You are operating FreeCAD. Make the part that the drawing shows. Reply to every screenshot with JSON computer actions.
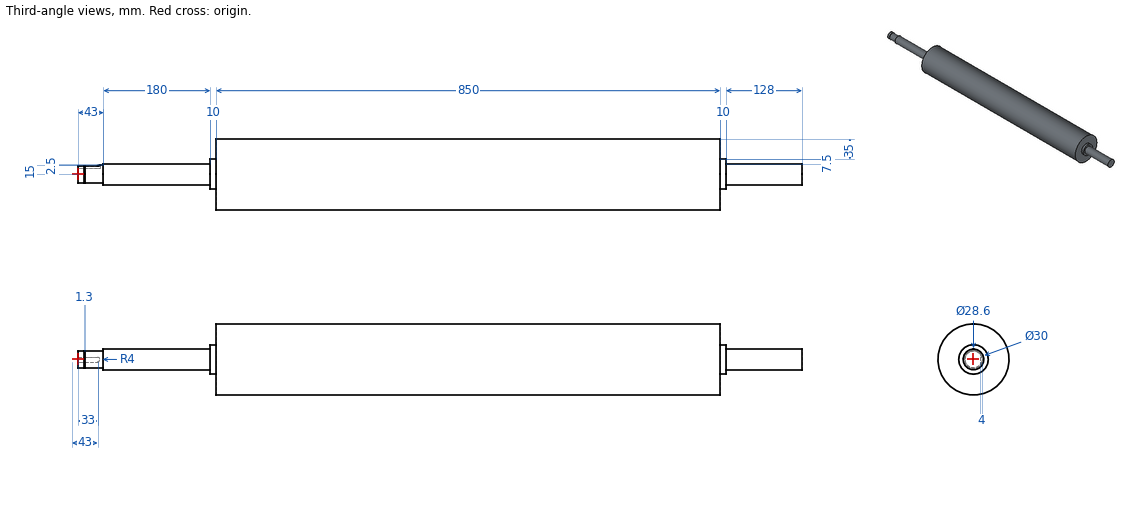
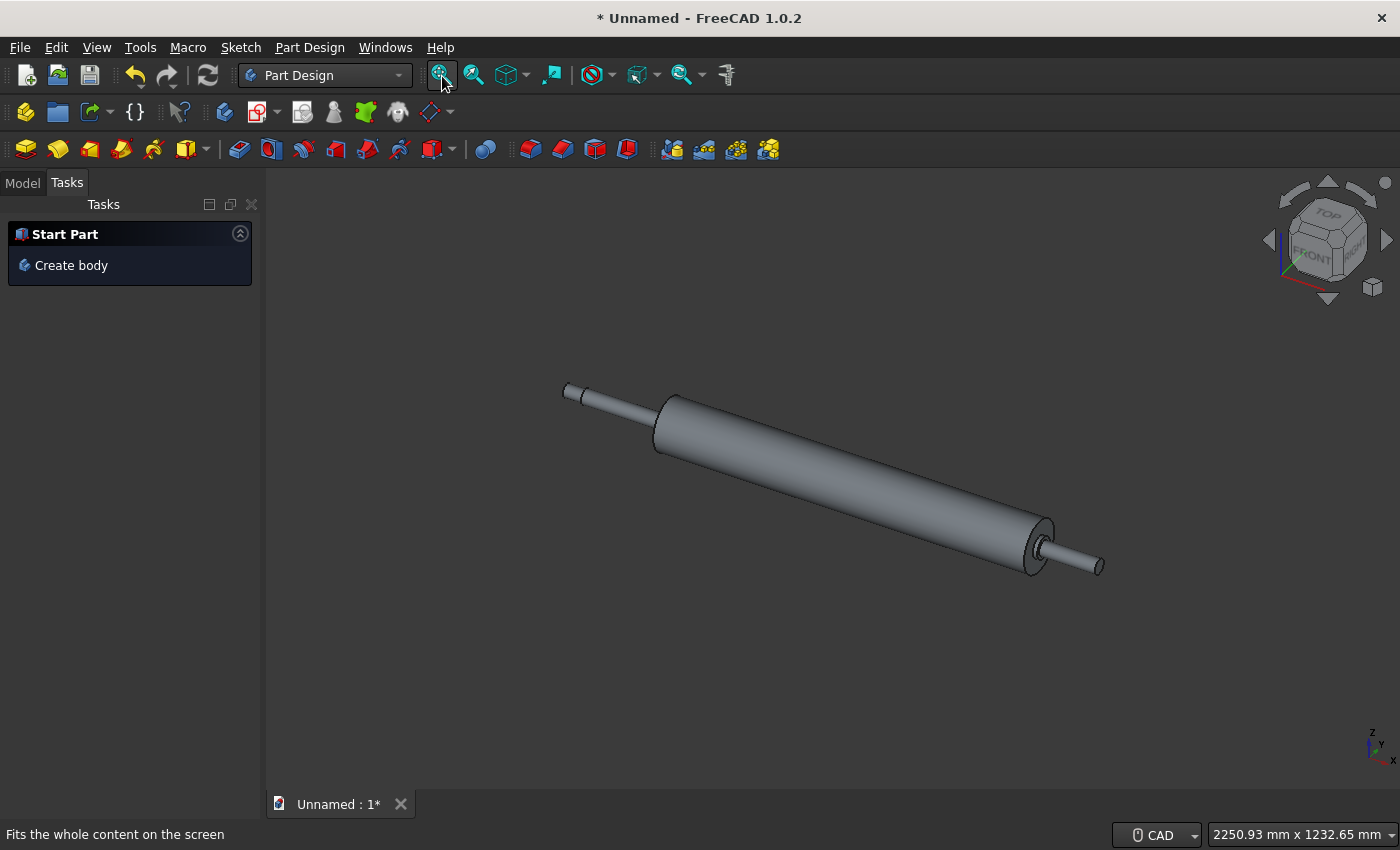
{"action": "left_click", "coordinate": [23, 182]}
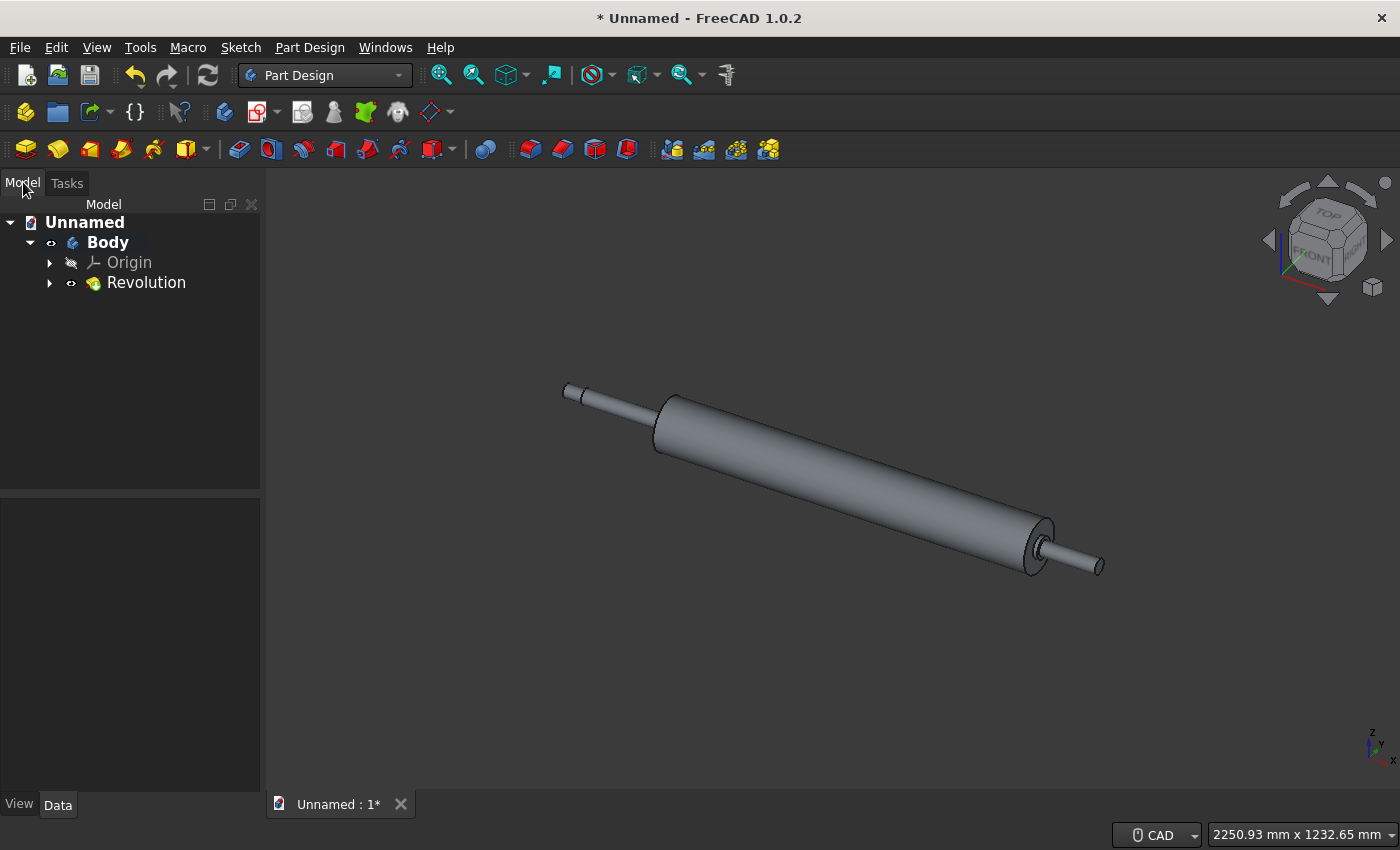
{"action": "left_click", "coordinate": [50, 263]}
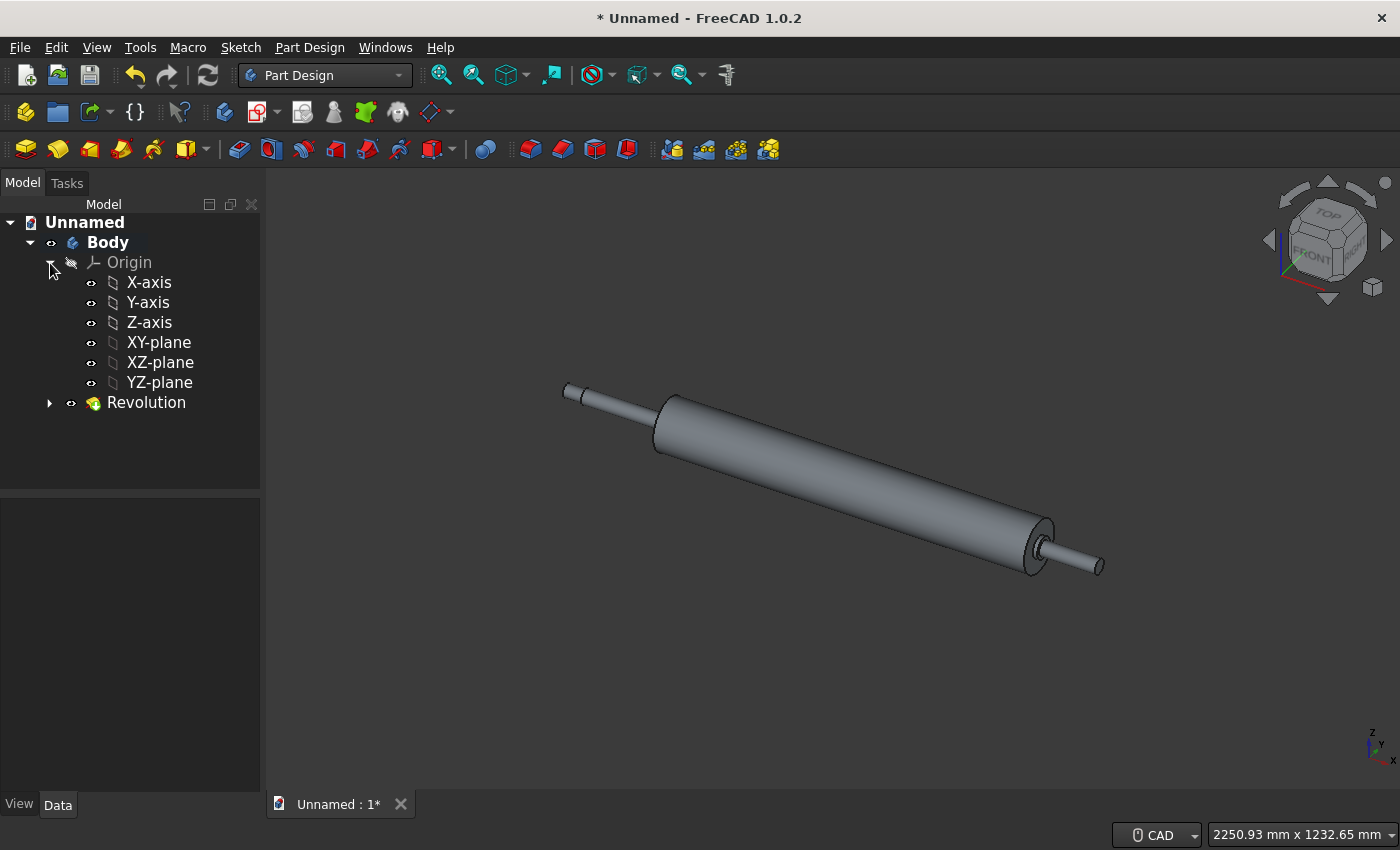
{"action": "left_click", "coordinate": [136, 363]}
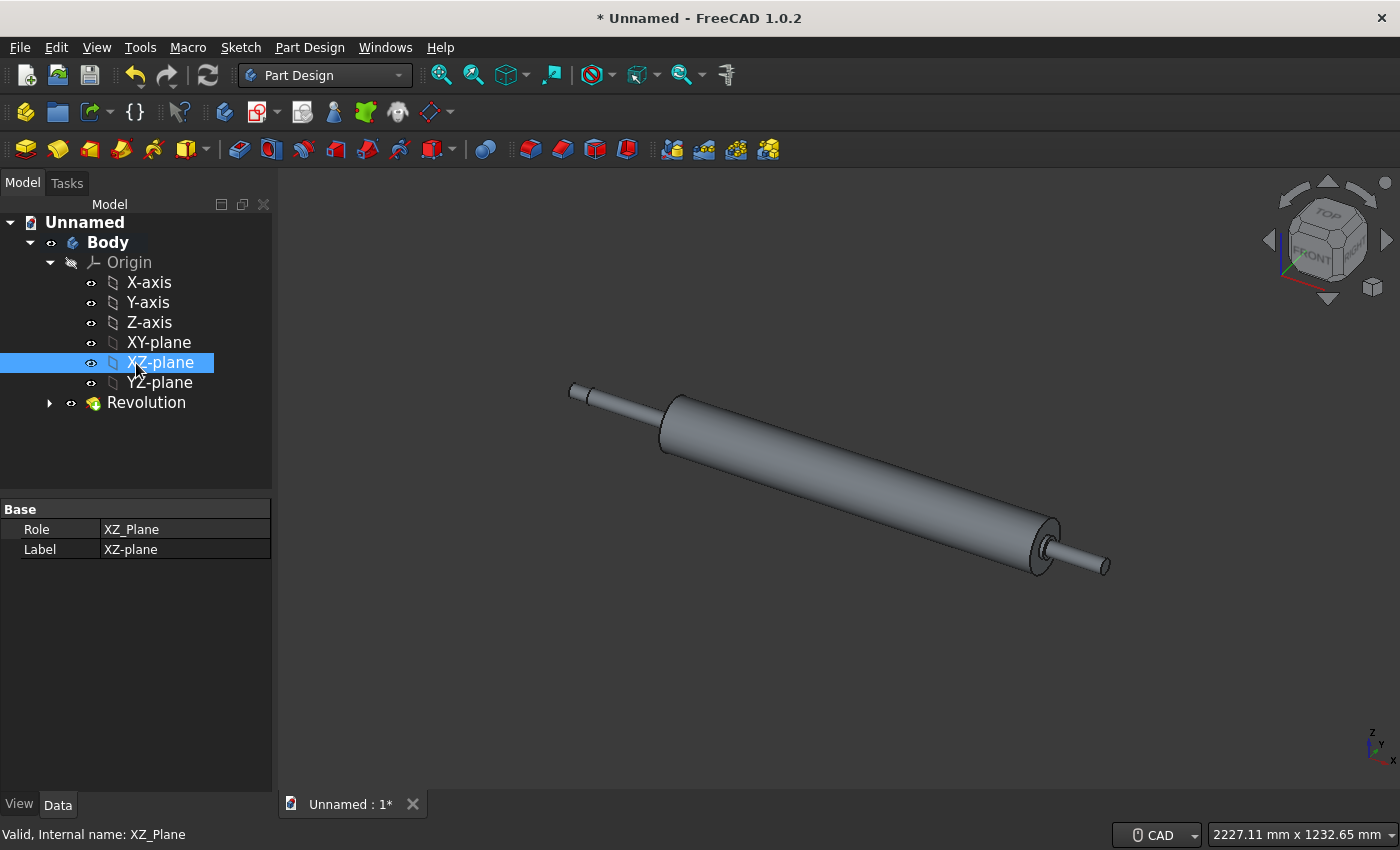
{"action": "left_click", "coordinate": [430, 112]}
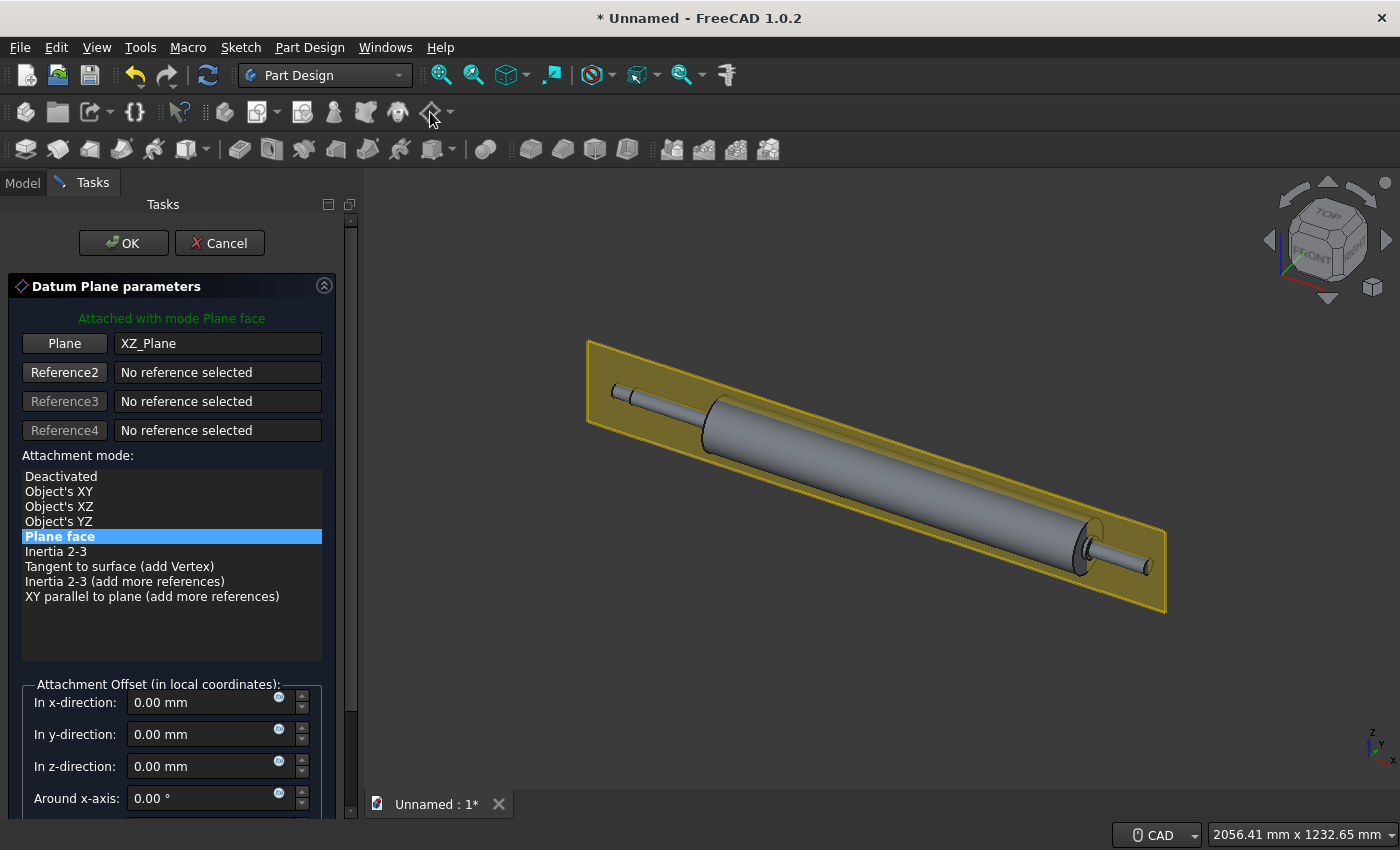
{"action": "triple_click", "coordinate": [210, 766]}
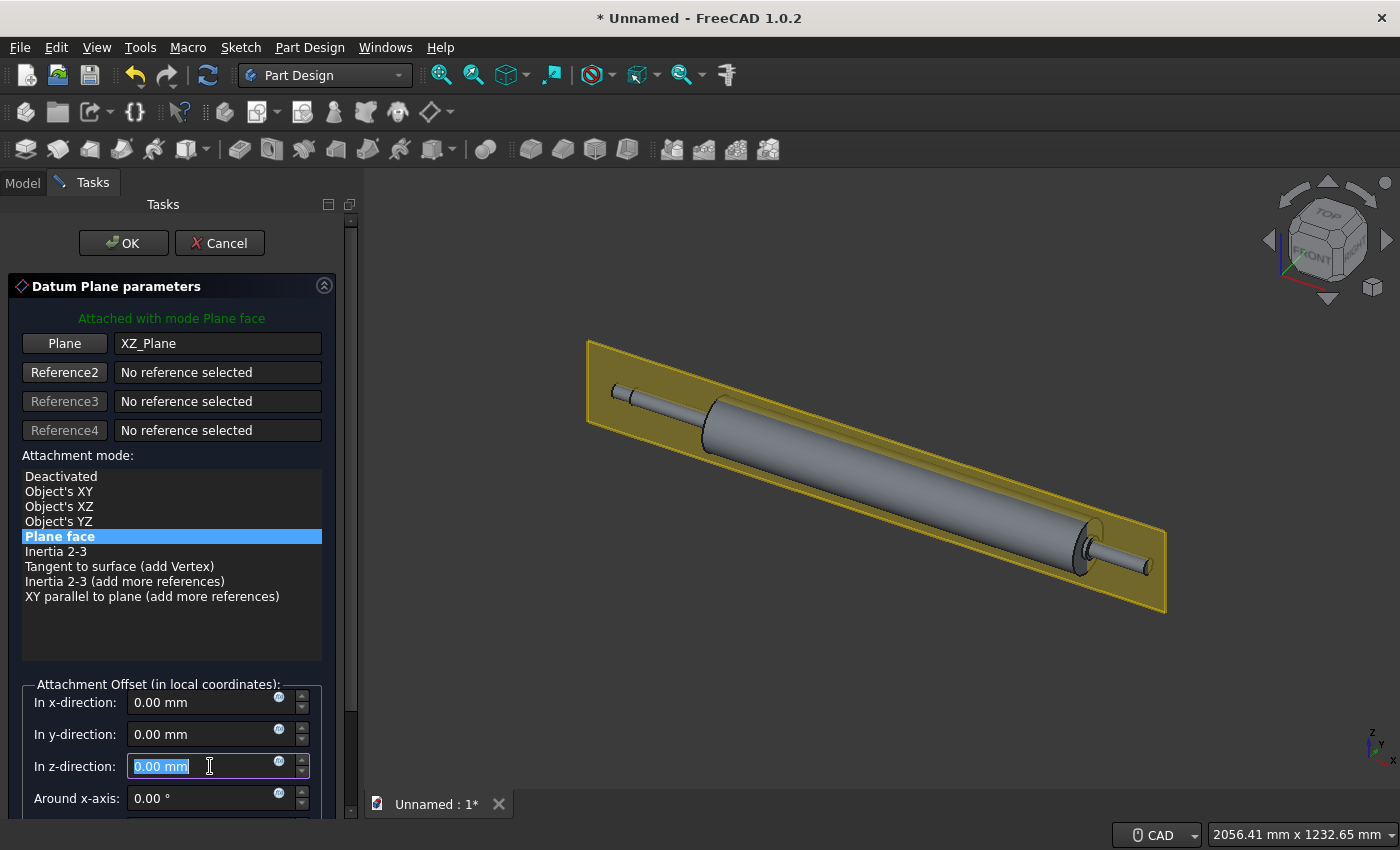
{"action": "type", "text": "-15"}
{"action": "key", "text": "Tab"}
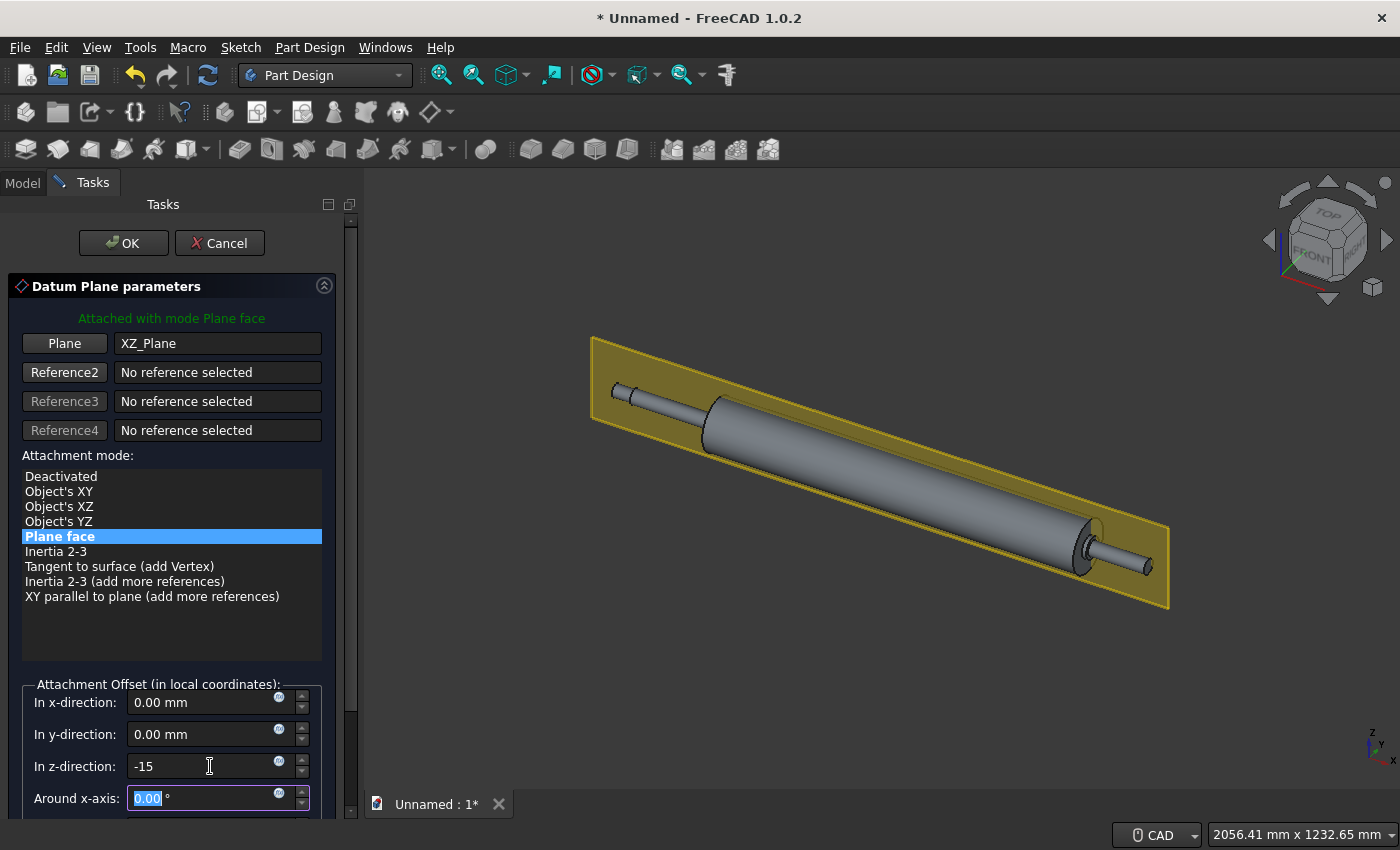
{"action": "left_click", "coordinate": [124, 243]}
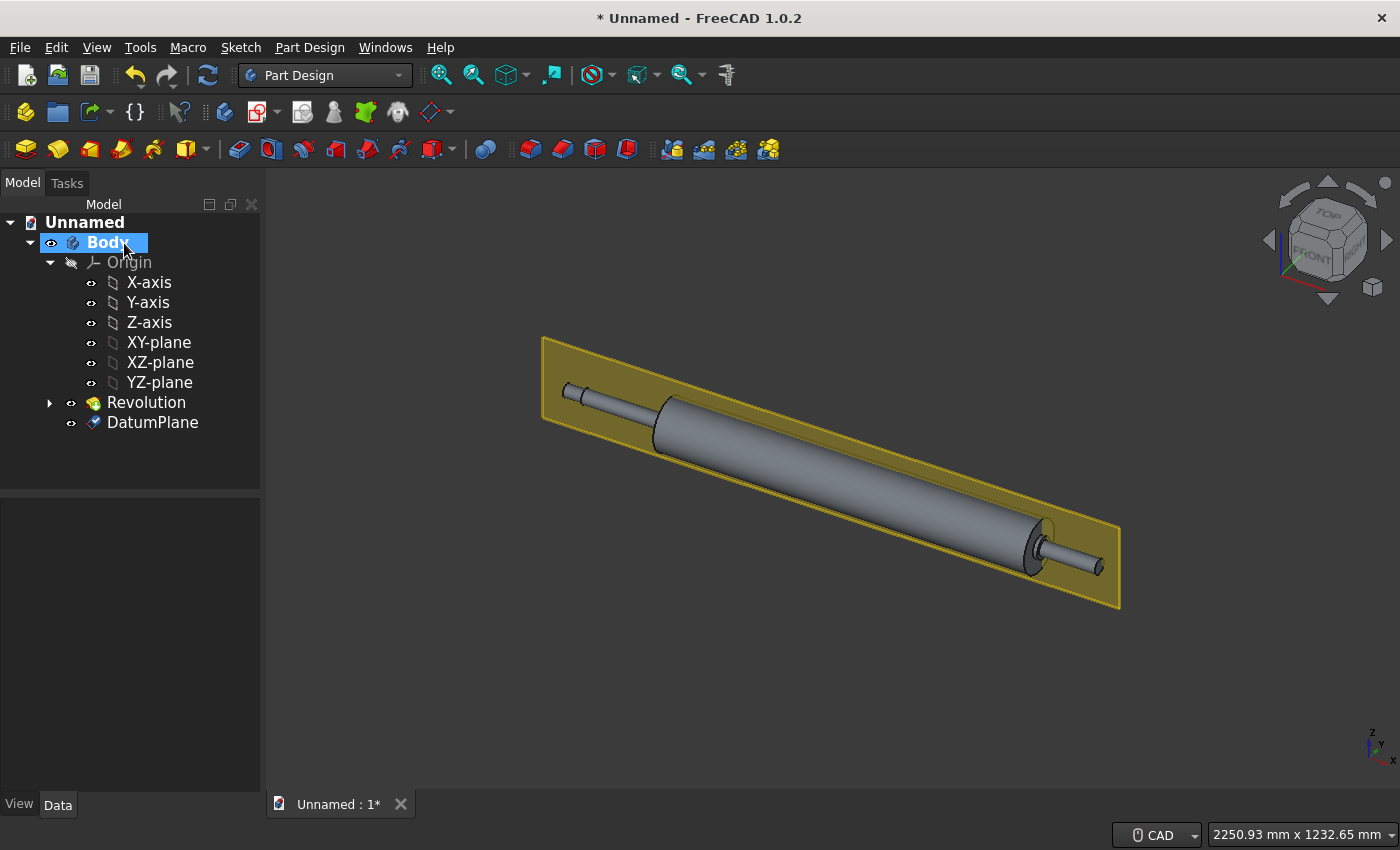
{"action": "left_click", "coordinate": [116, 423]}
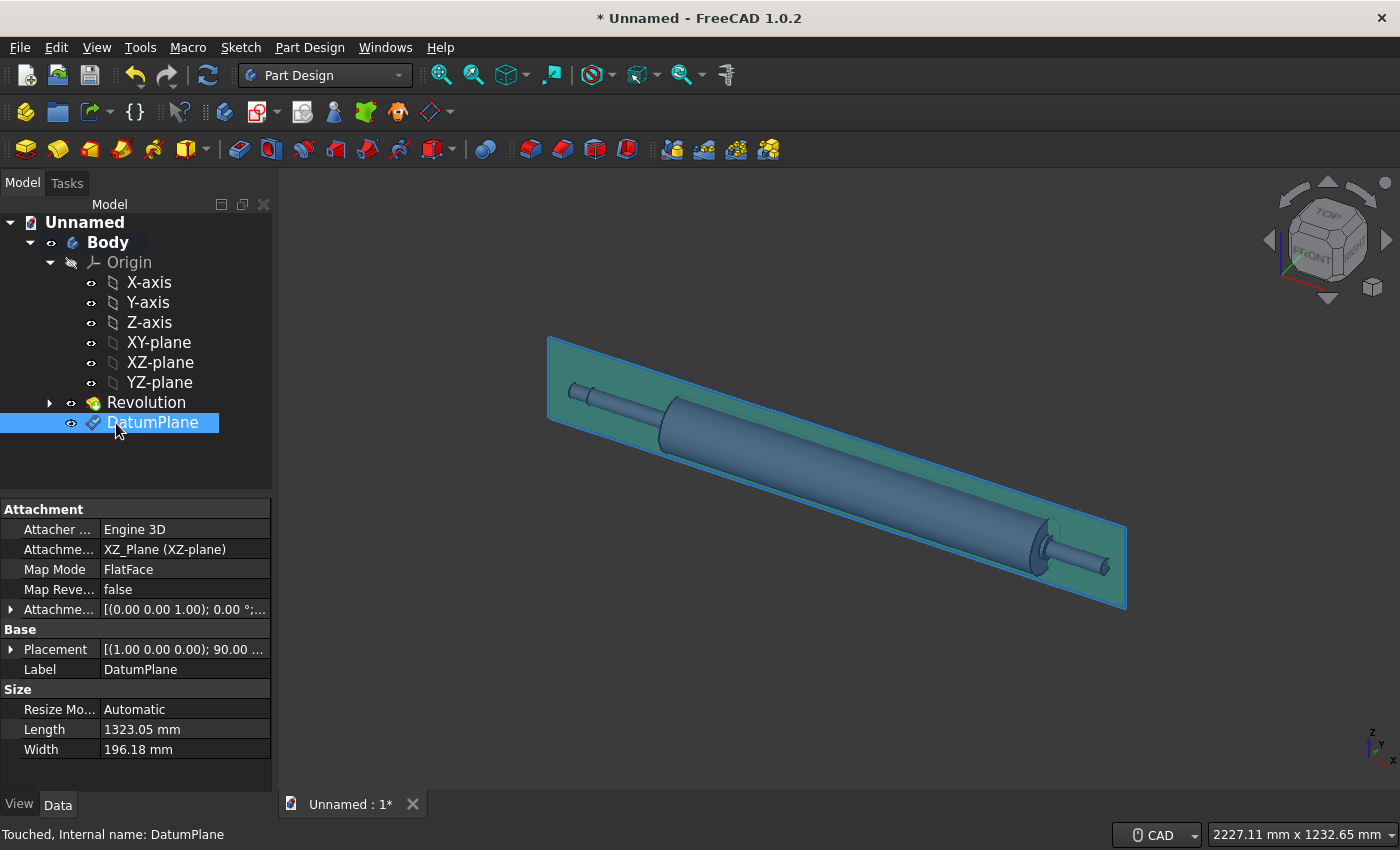
{"action": "left_click", "coordinate": [258, 112]}